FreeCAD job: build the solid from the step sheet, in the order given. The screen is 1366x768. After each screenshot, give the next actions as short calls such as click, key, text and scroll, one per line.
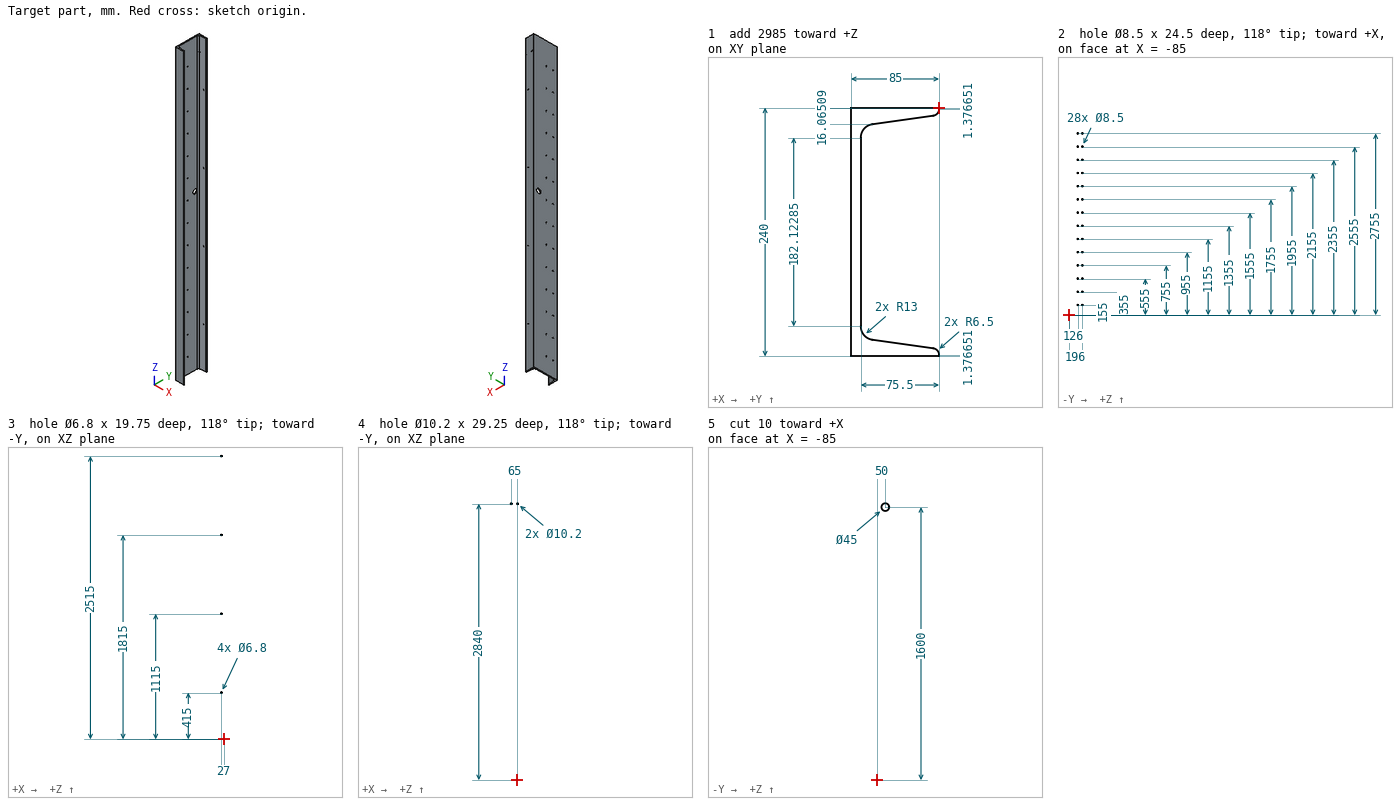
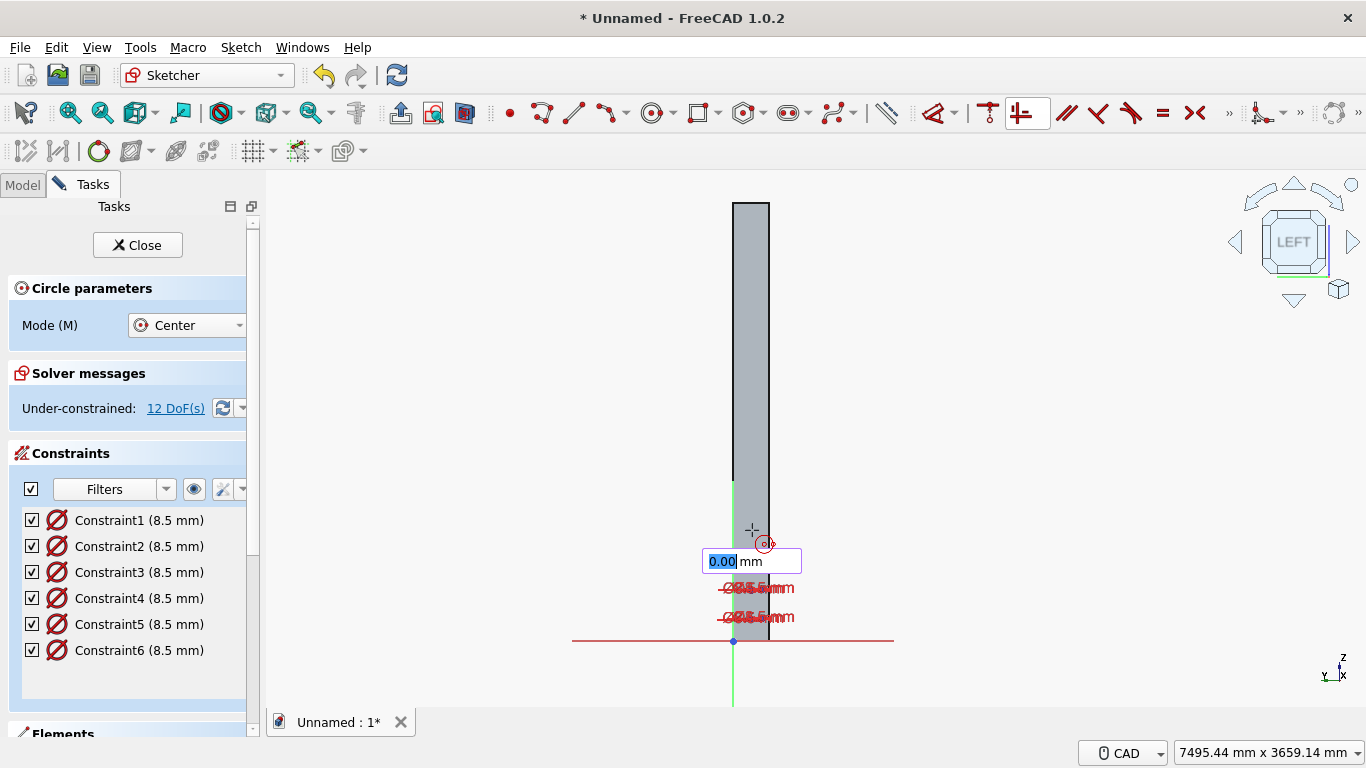
text(8.5)
key(Return)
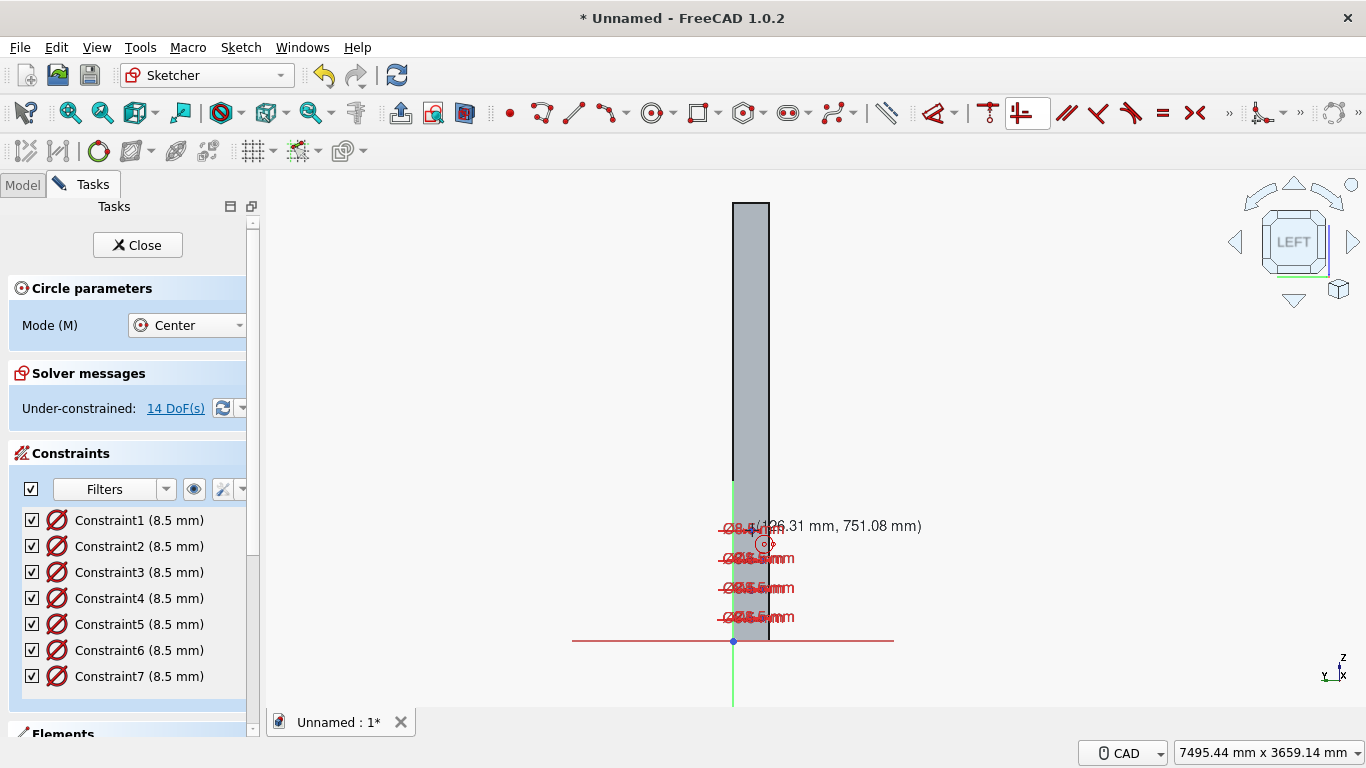
scroll(762, 530, up, 18)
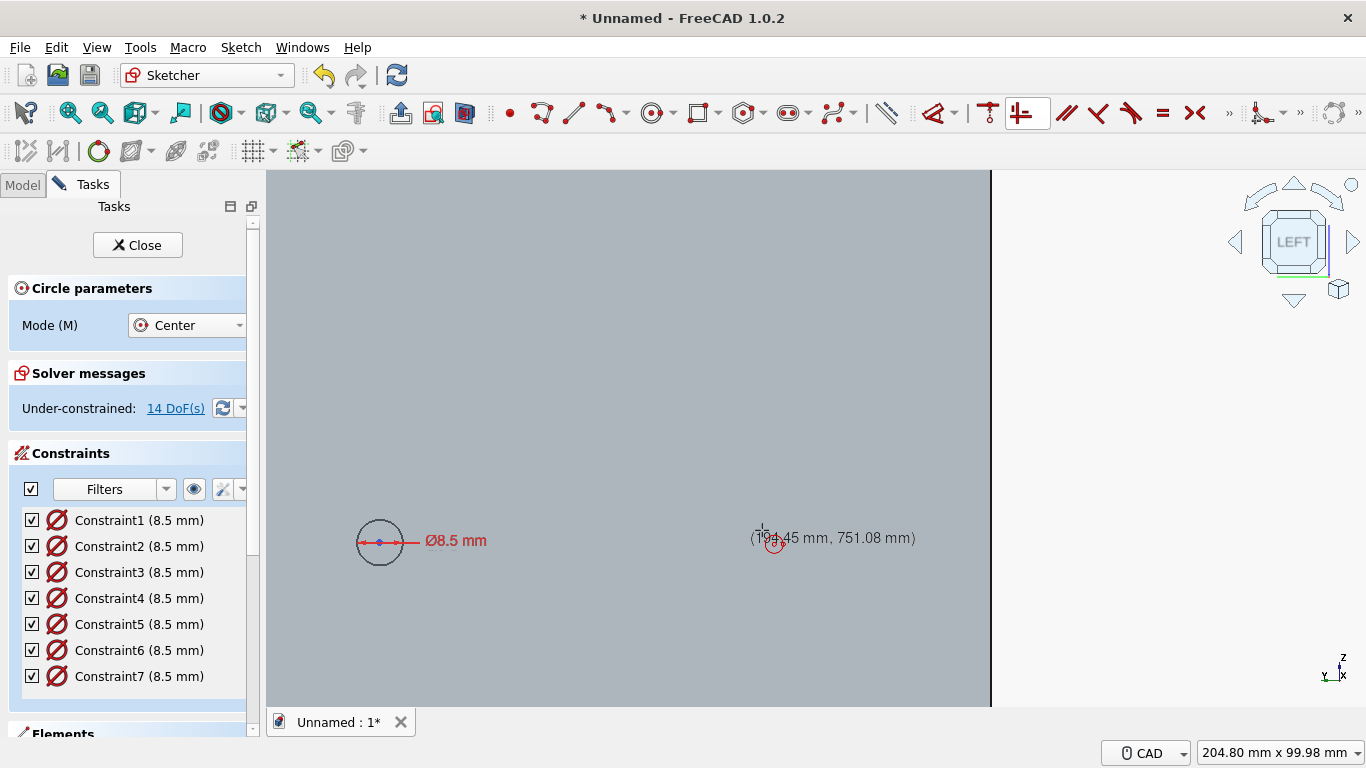
scroll(762, 530, down, 18)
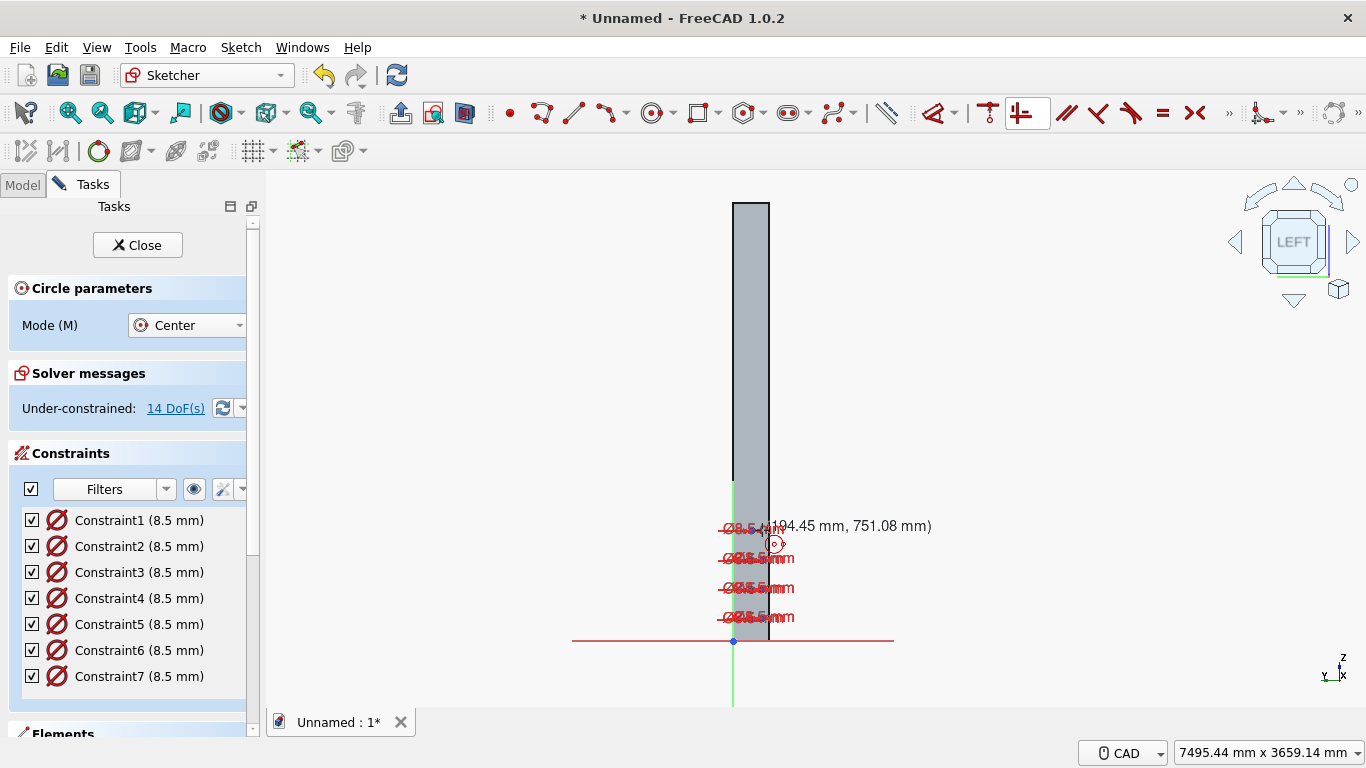
scroll(762, 530, up, 3)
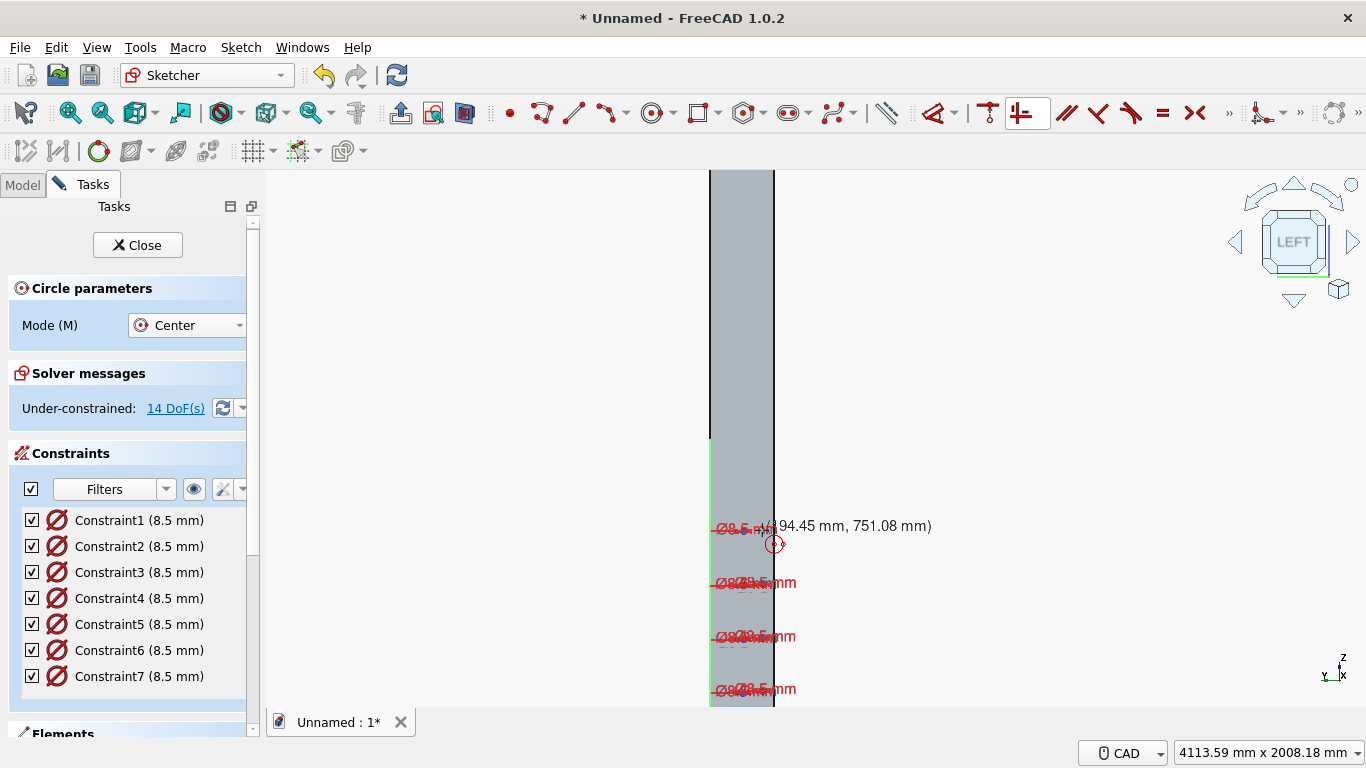
click(762, 530)
move(763, 529)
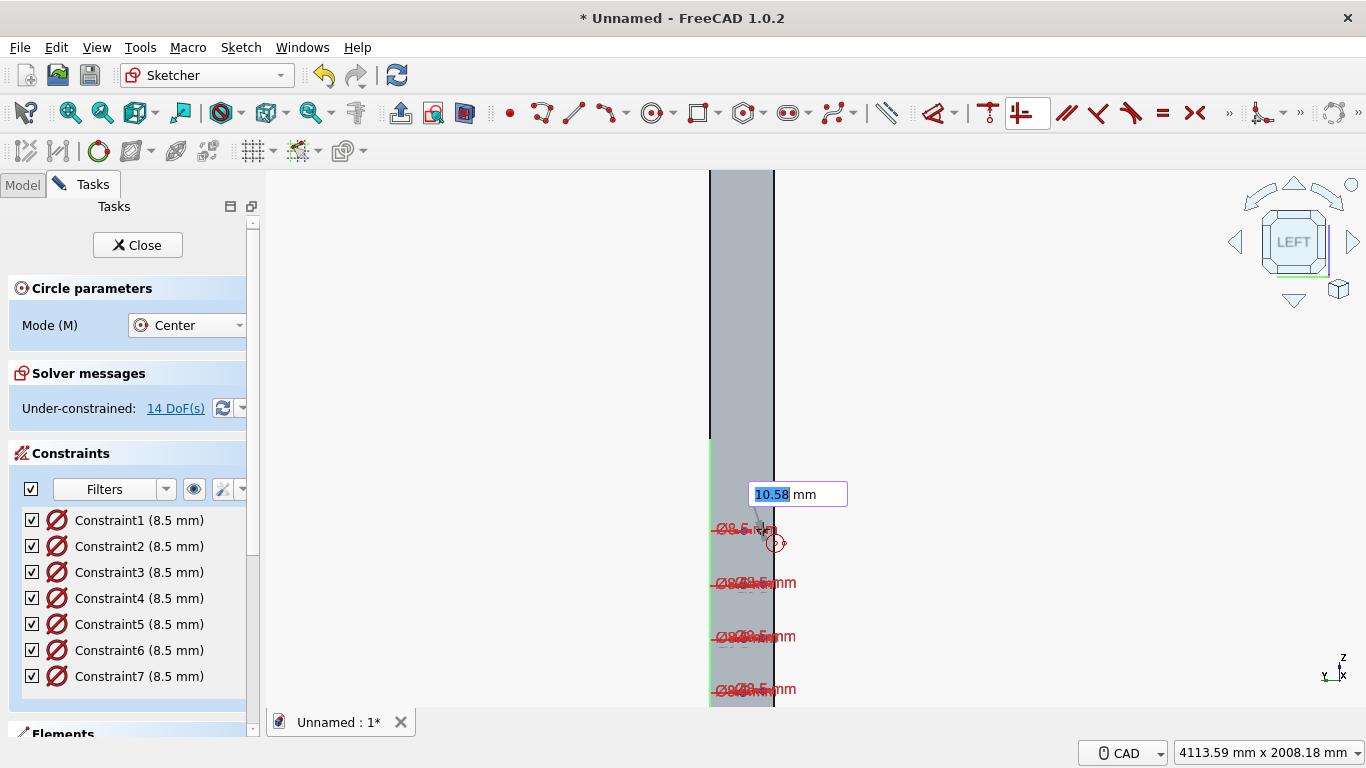
text(8.5)
key(Return)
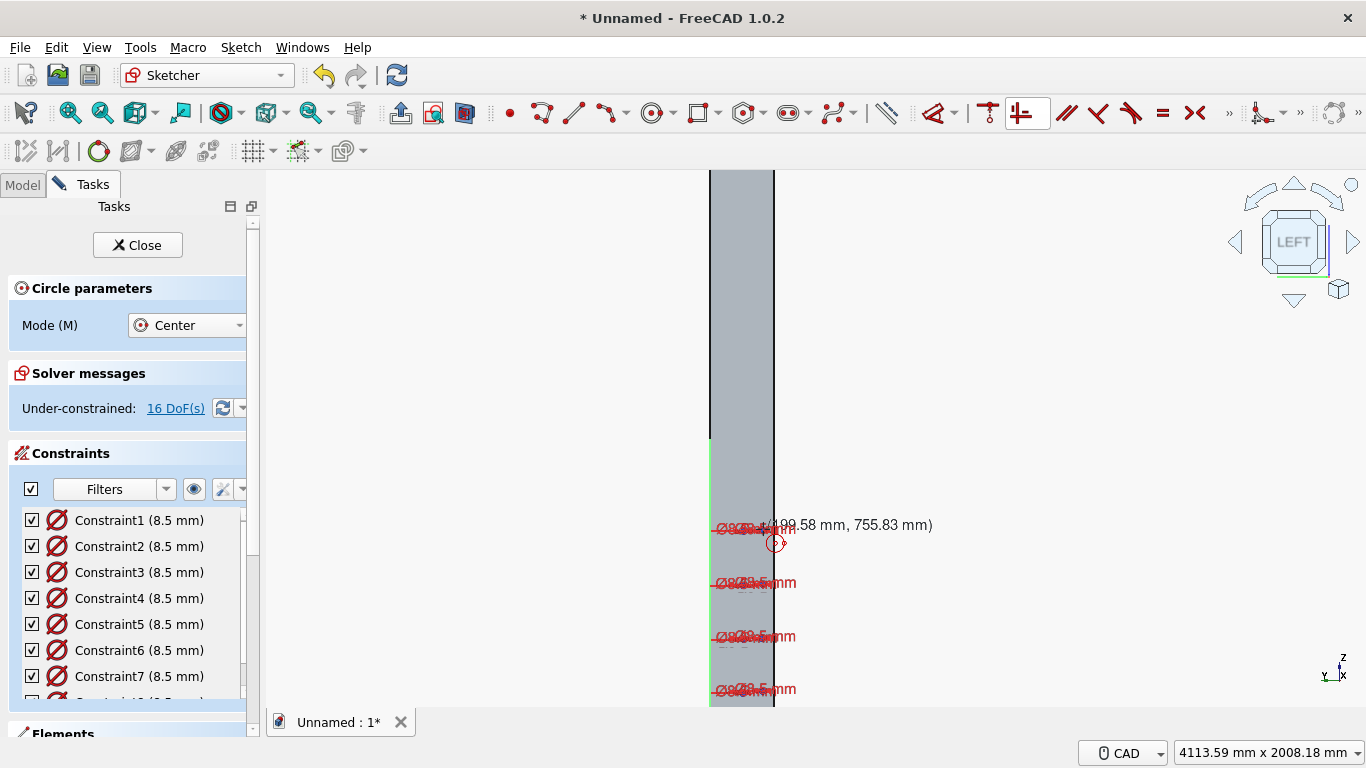
scroll(743, 477, up, 15)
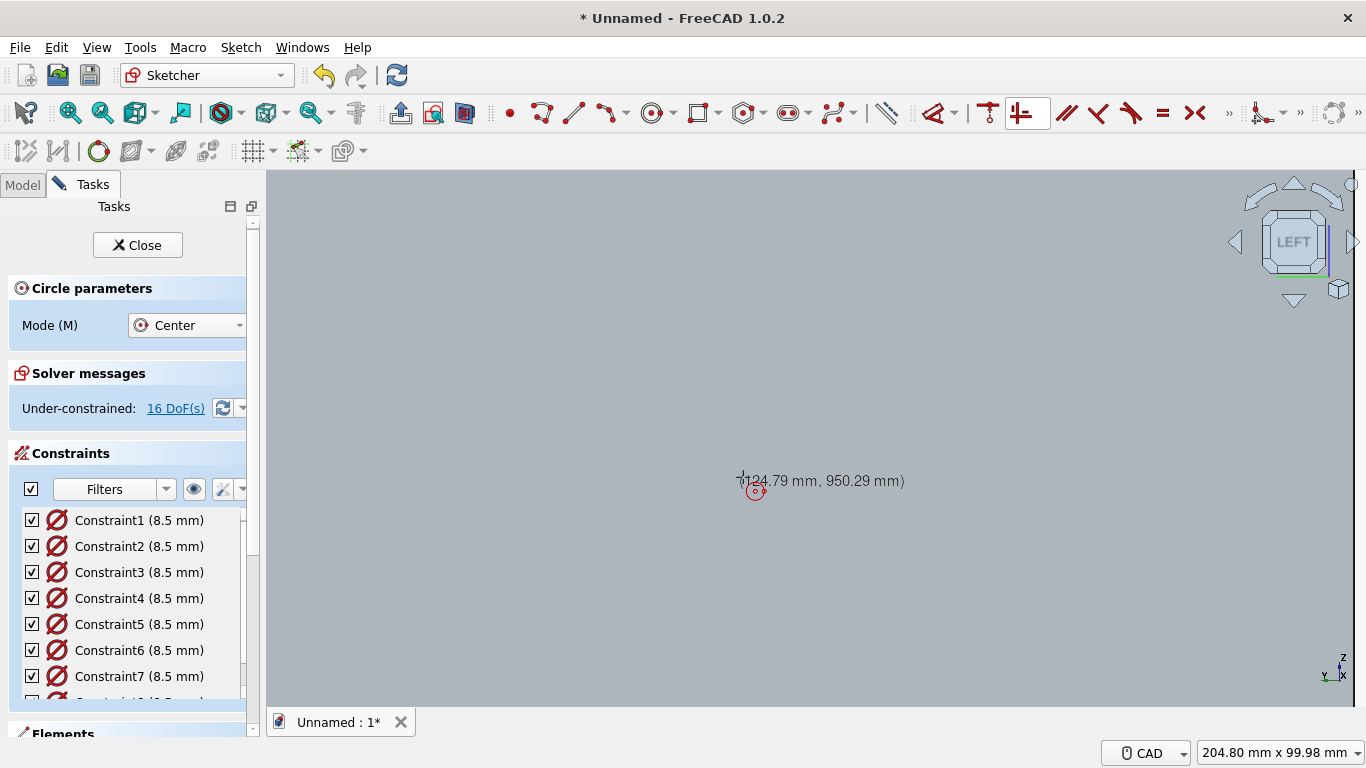
scroll(752, 502, down, 18)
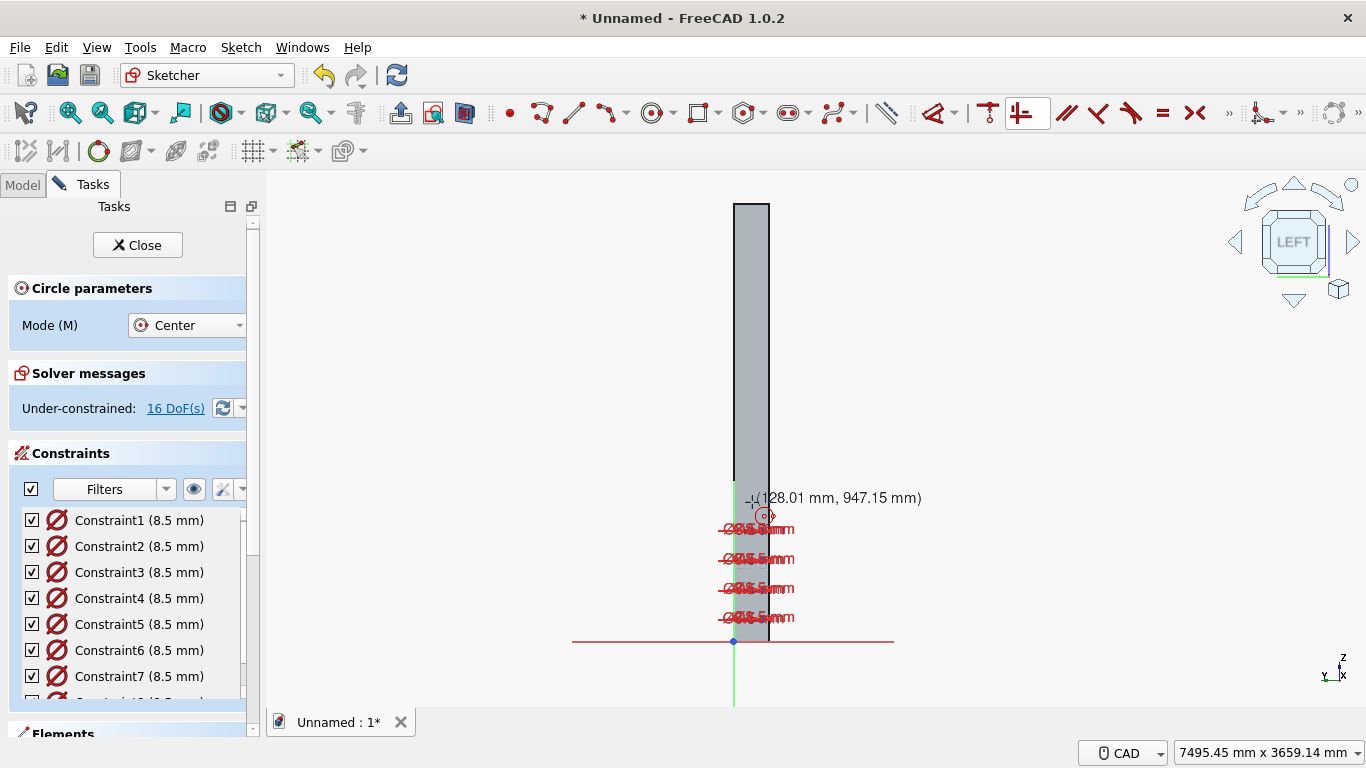
click(752, 501)
move(753, 501)